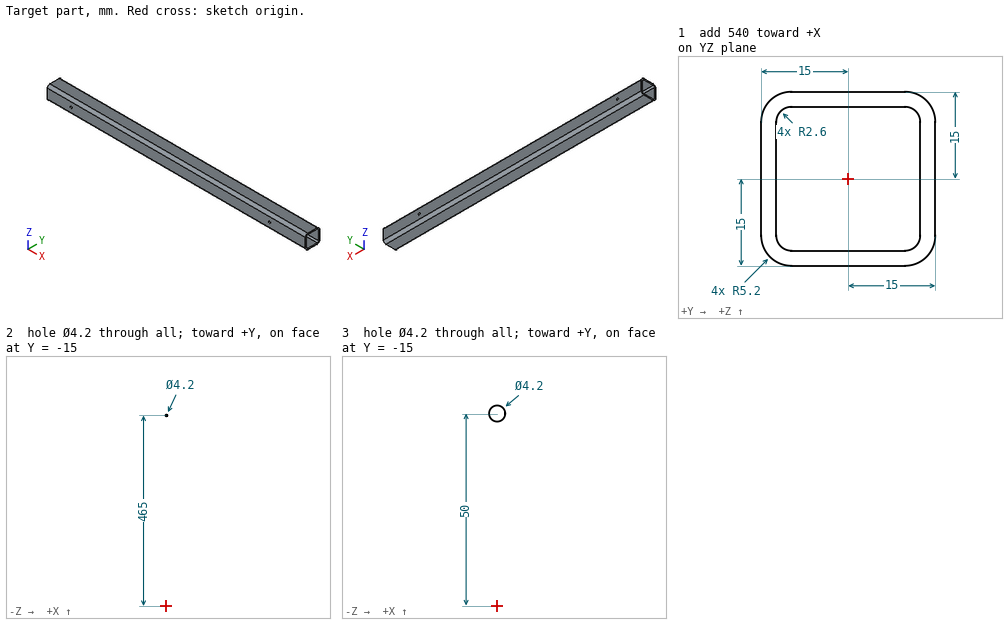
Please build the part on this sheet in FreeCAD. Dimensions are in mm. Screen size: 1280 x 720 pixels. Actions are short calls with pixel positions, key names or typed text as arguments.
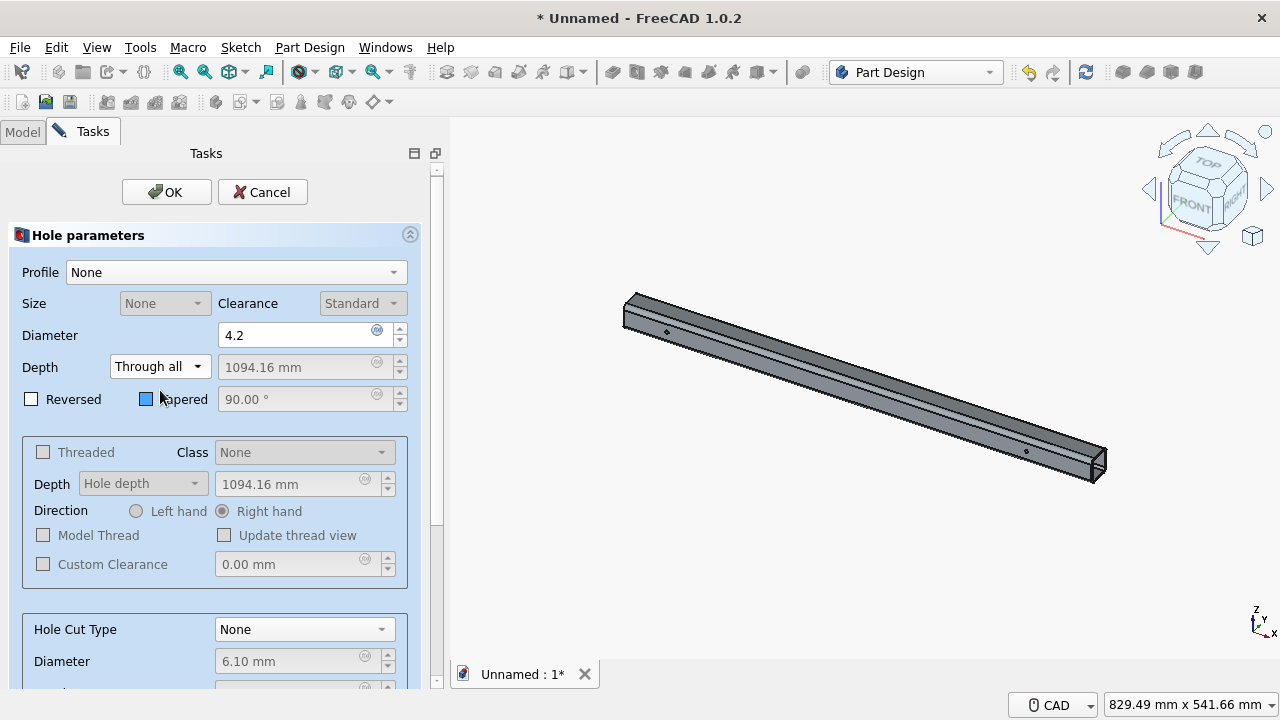
click(167, 192)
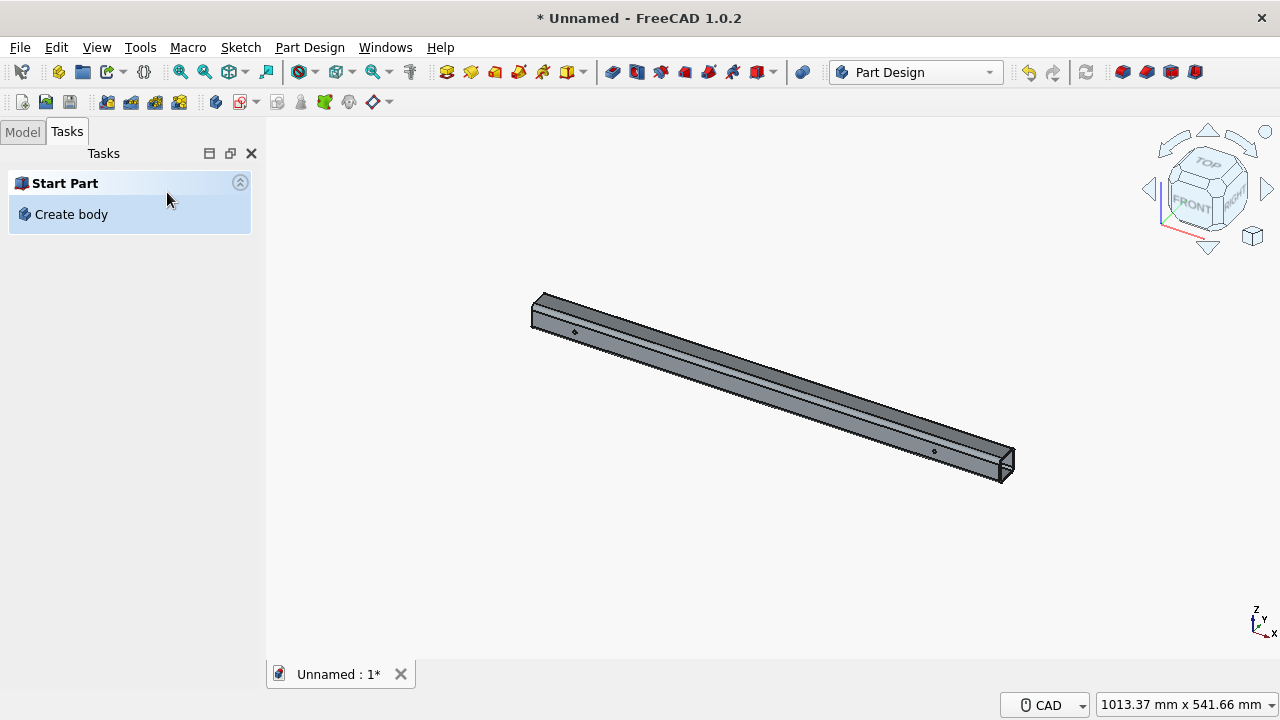
key(0)